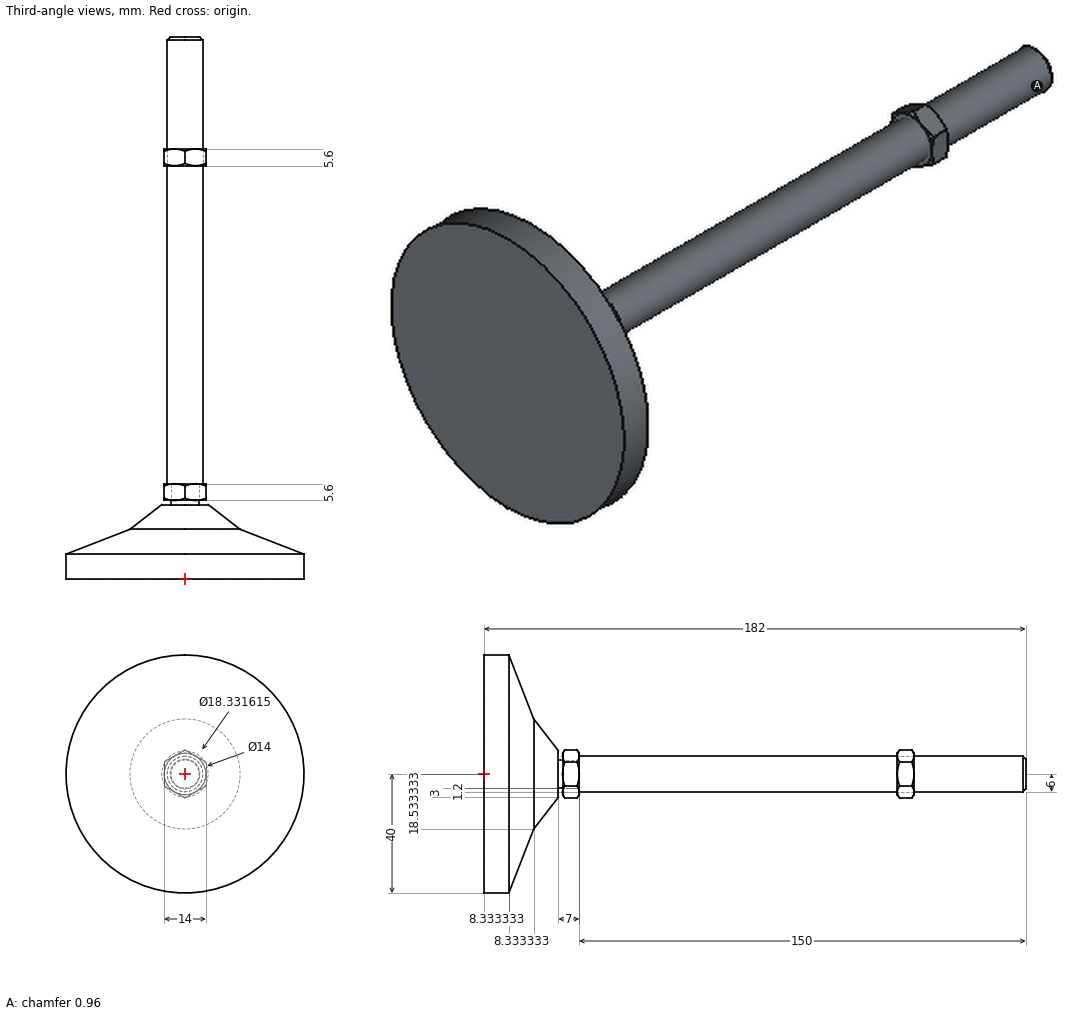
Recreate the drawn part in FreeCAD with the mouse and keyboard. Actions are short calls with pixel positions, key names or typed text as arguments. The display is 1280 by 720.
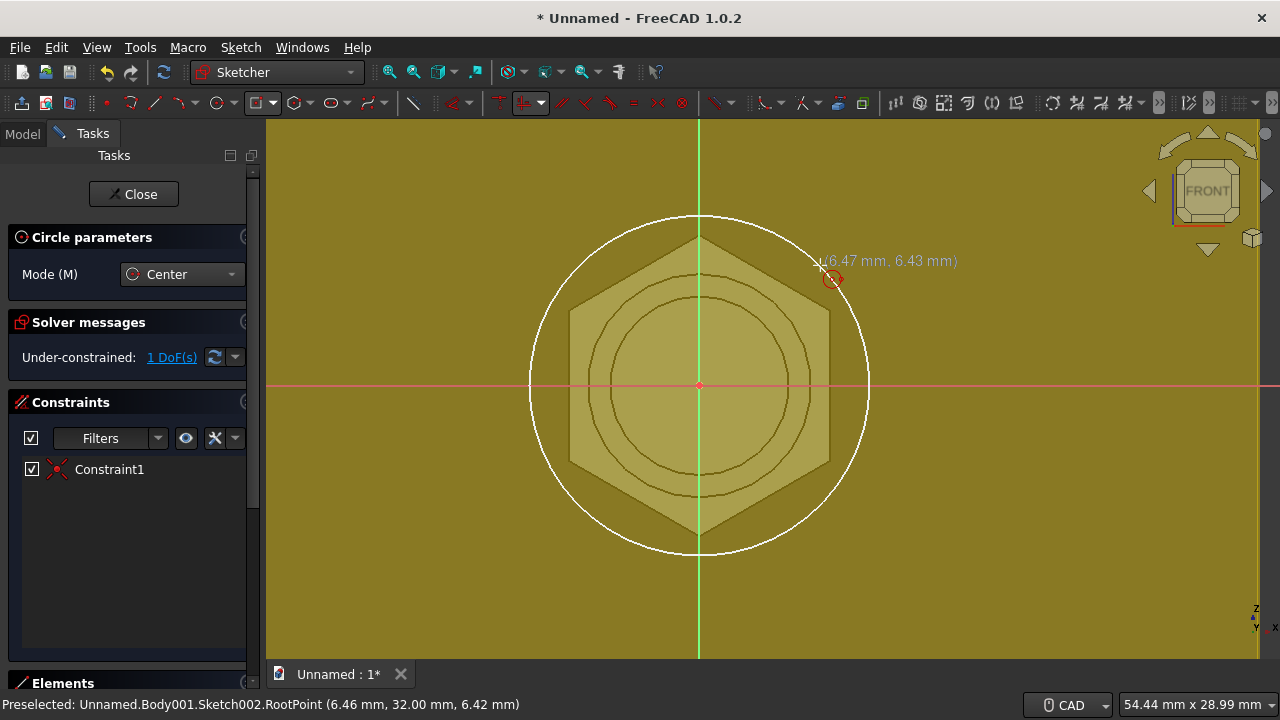
click(699, 386)
click(792, 294)
key(Escape)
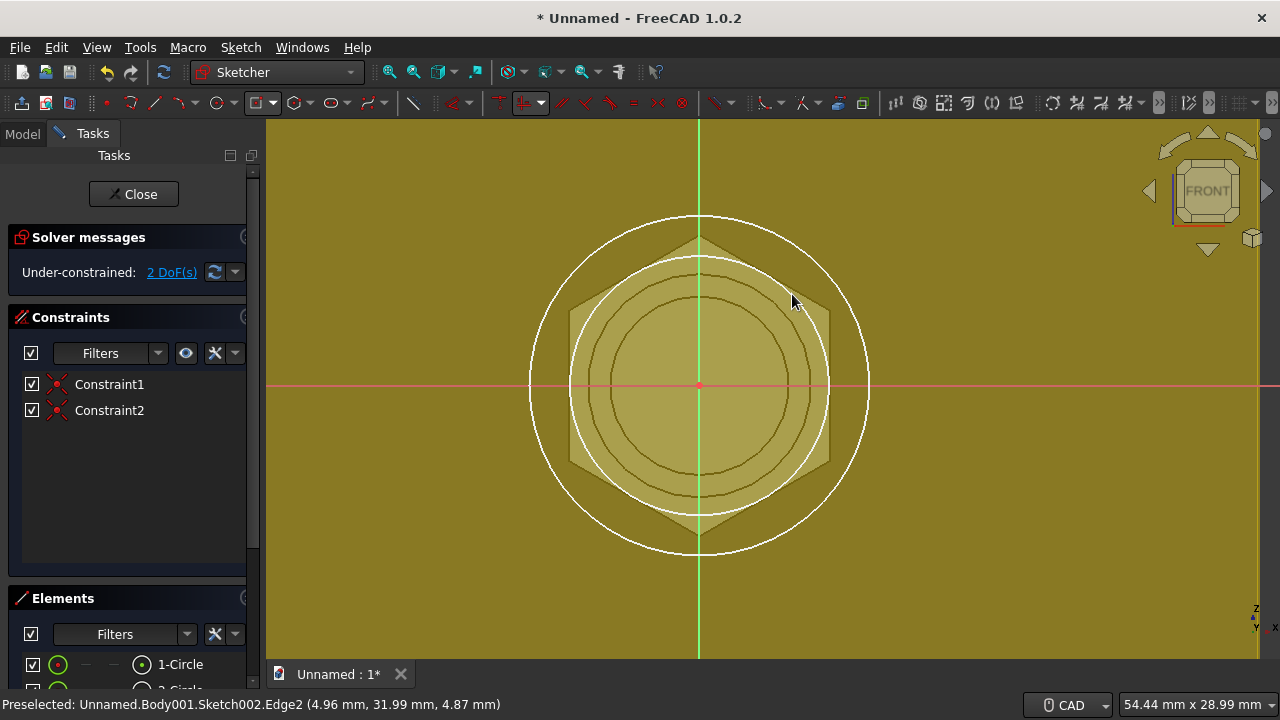
click(452, 104)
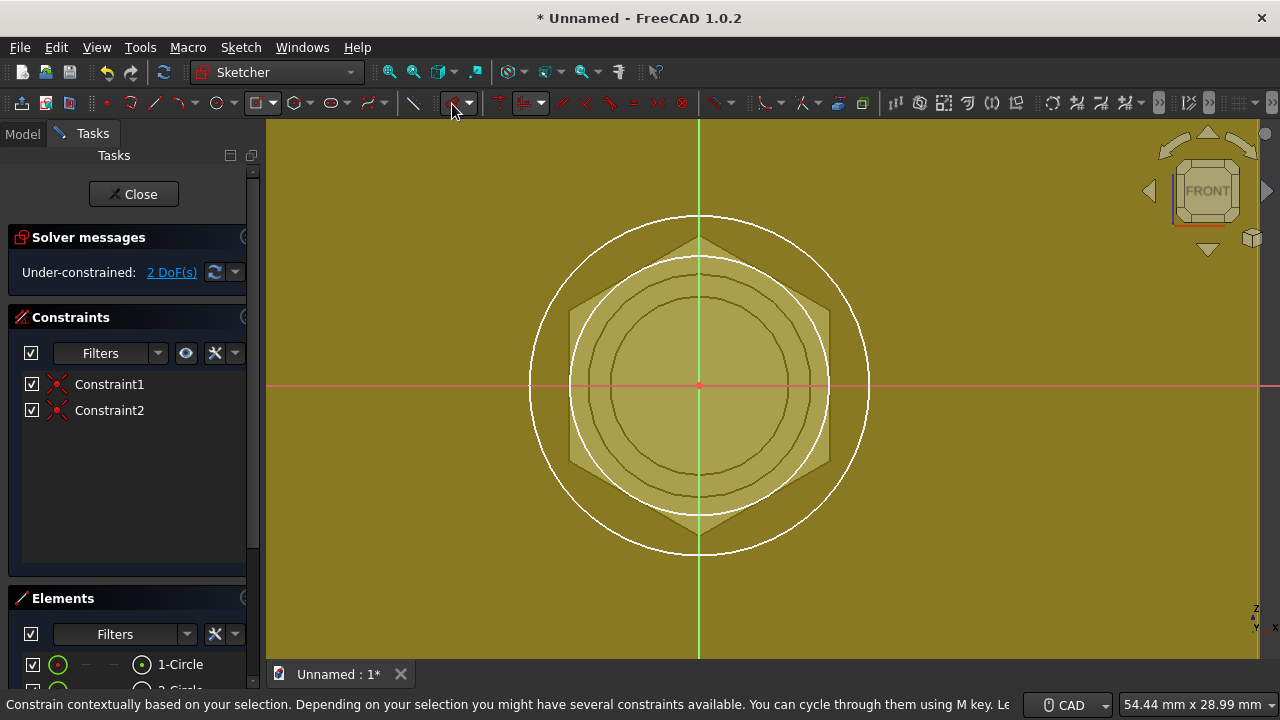
click(819, 265)
click(842, 242)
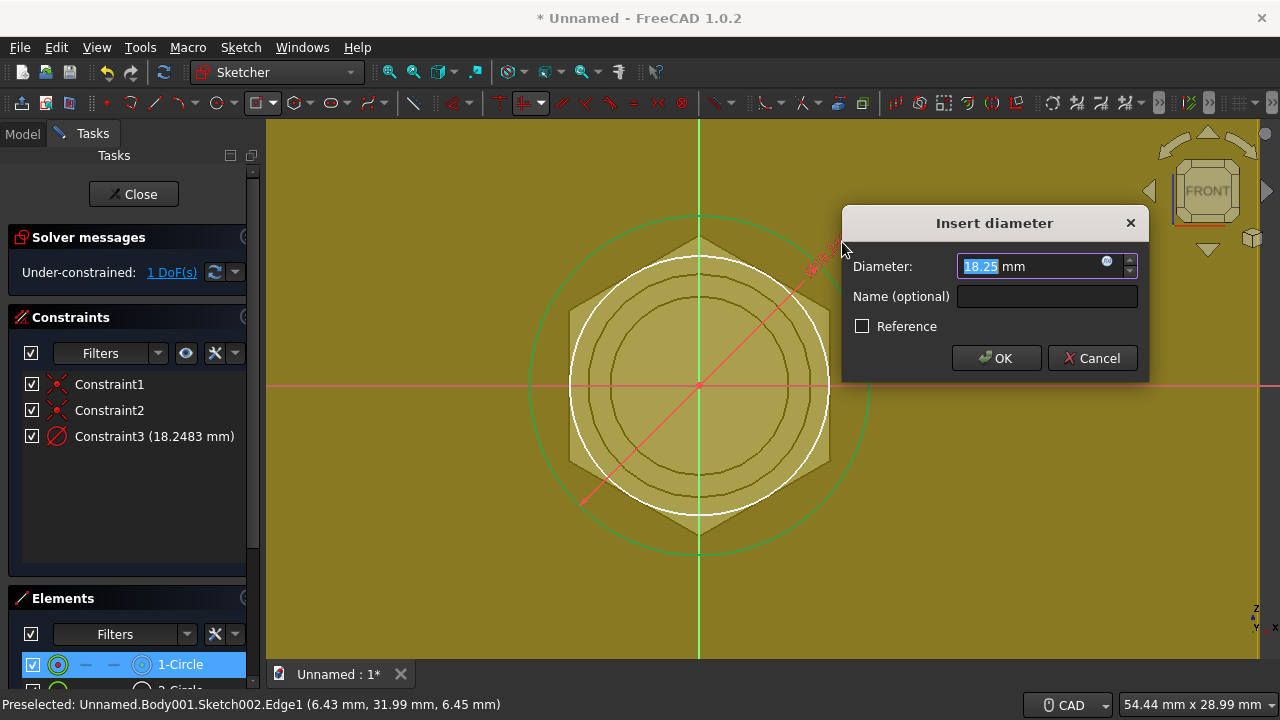
text(18.331615)
key(Return)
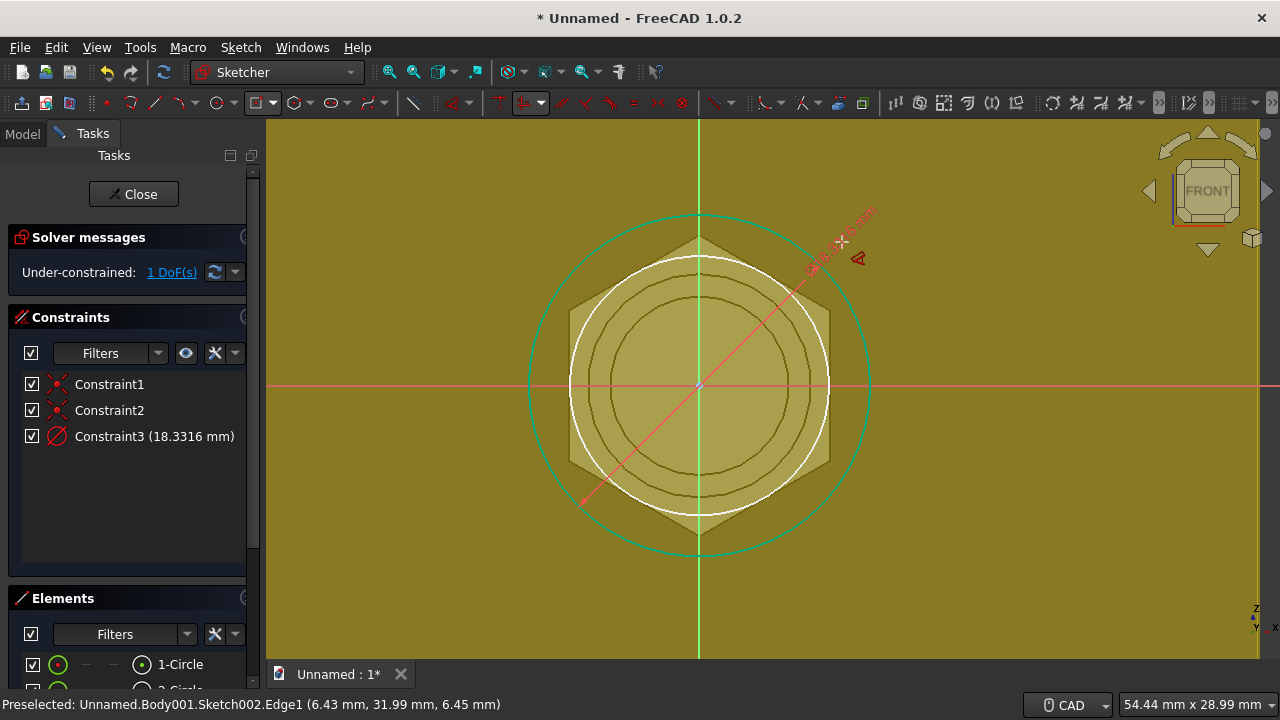
click(791, 294)
click(877, 334)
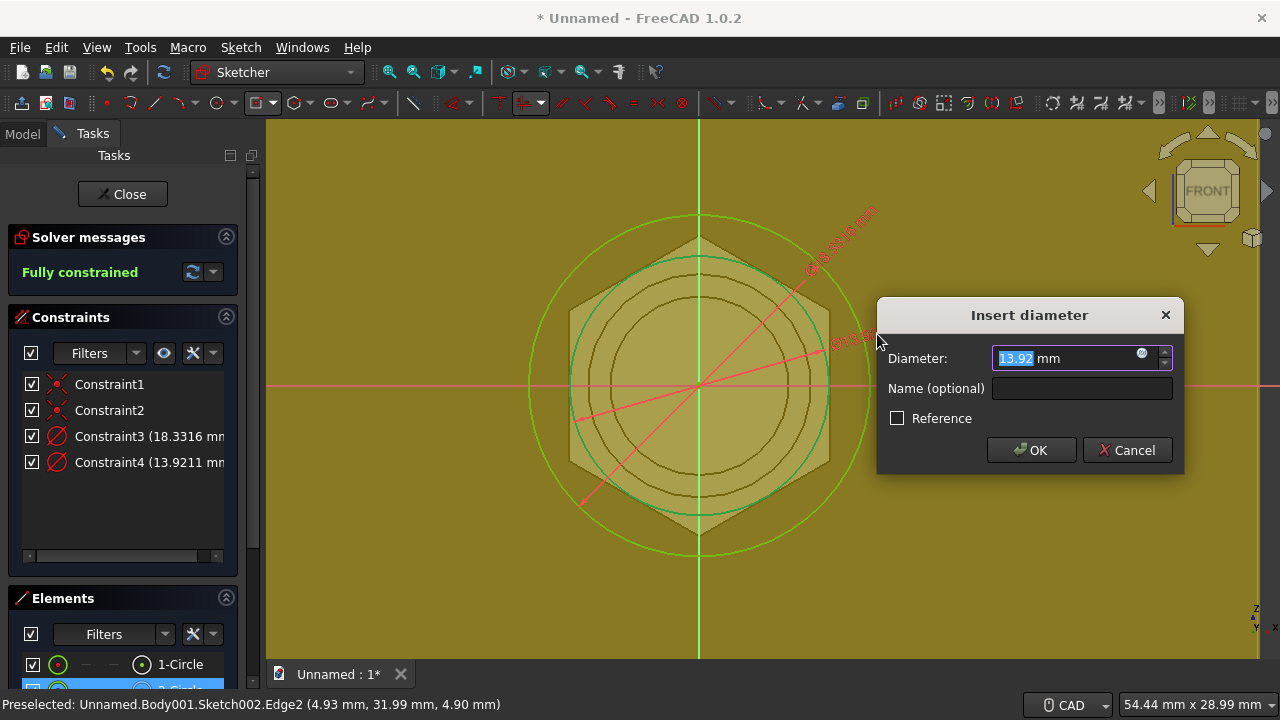
text(14)
key(Return)
key(Escape)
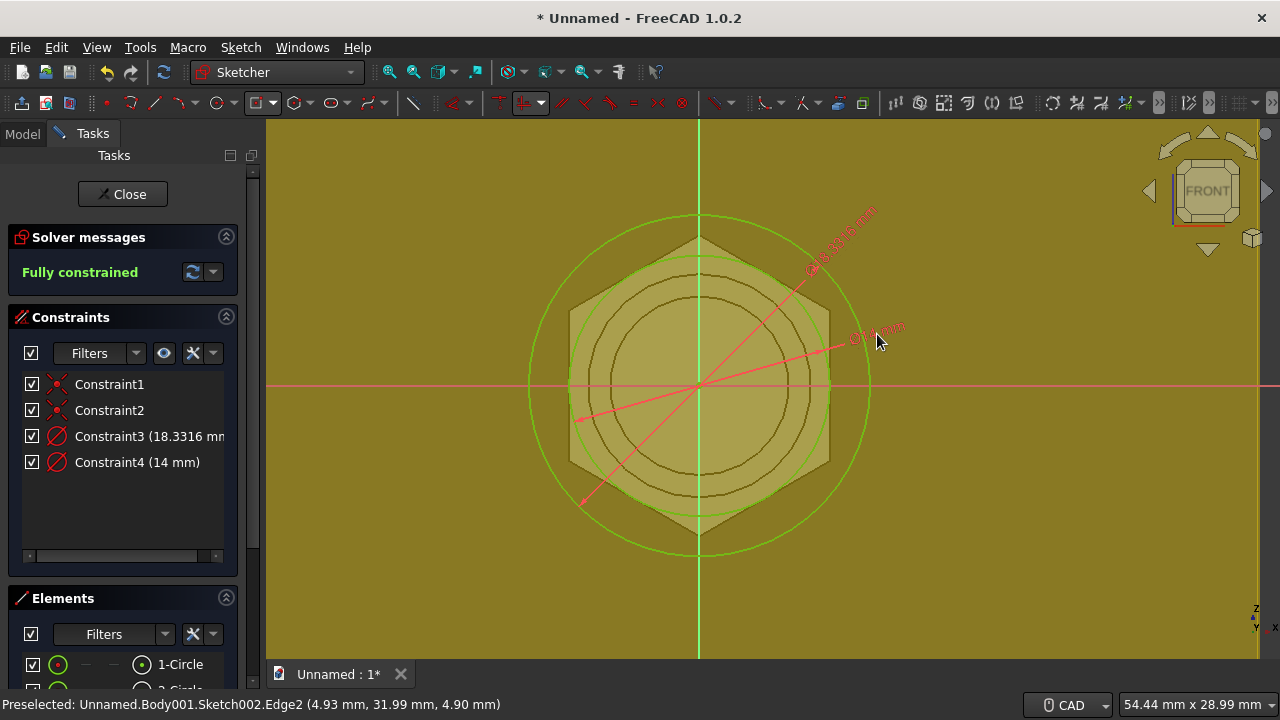
click(123, 194)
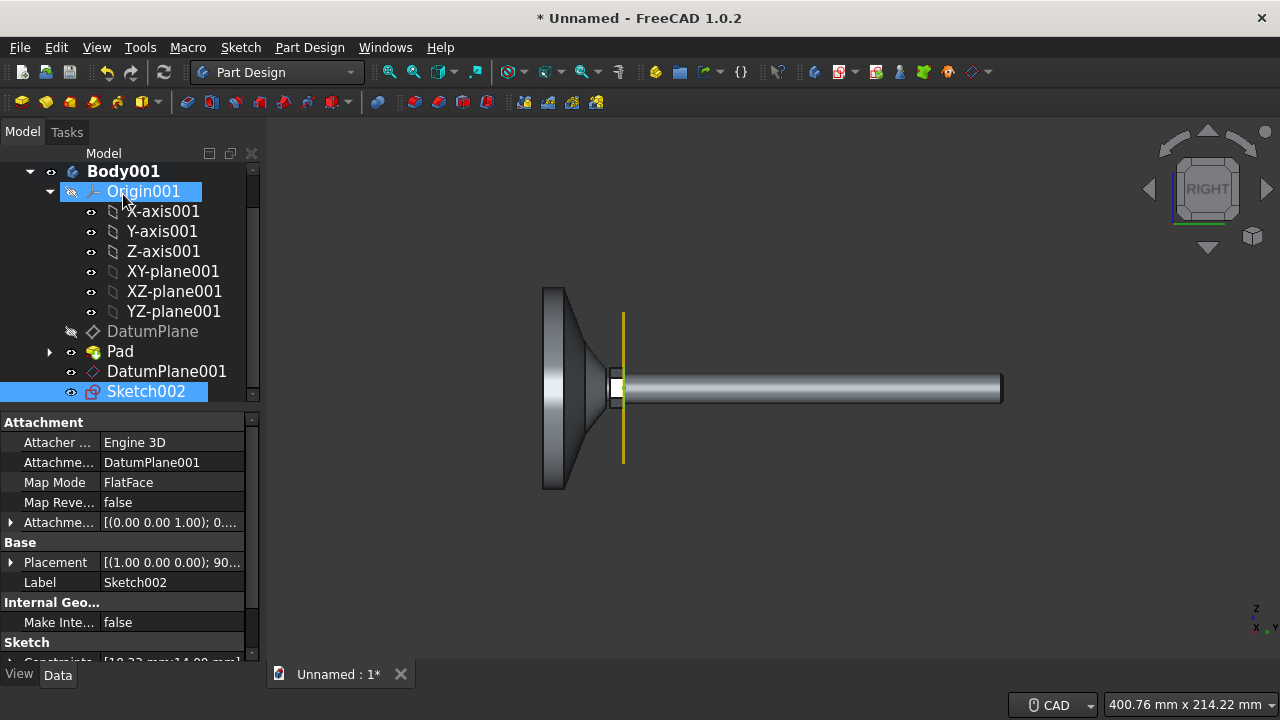
click(188, 102)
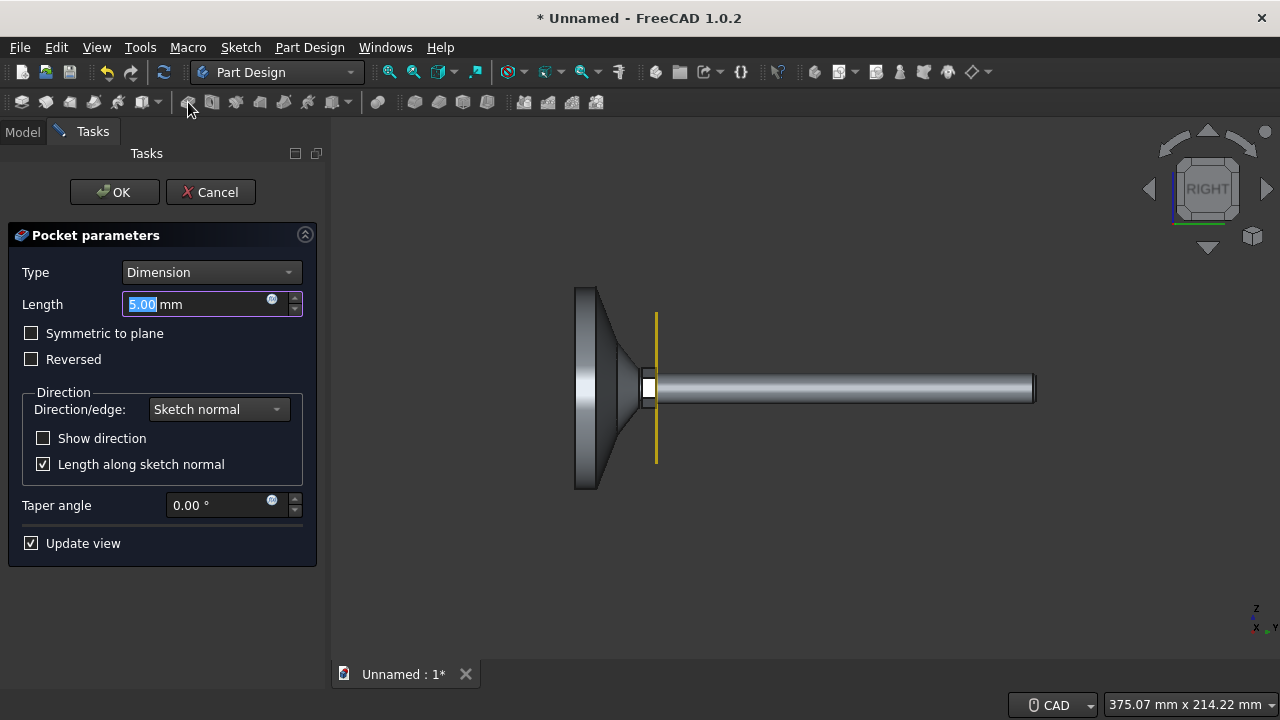
text(5.6)
key(Tab)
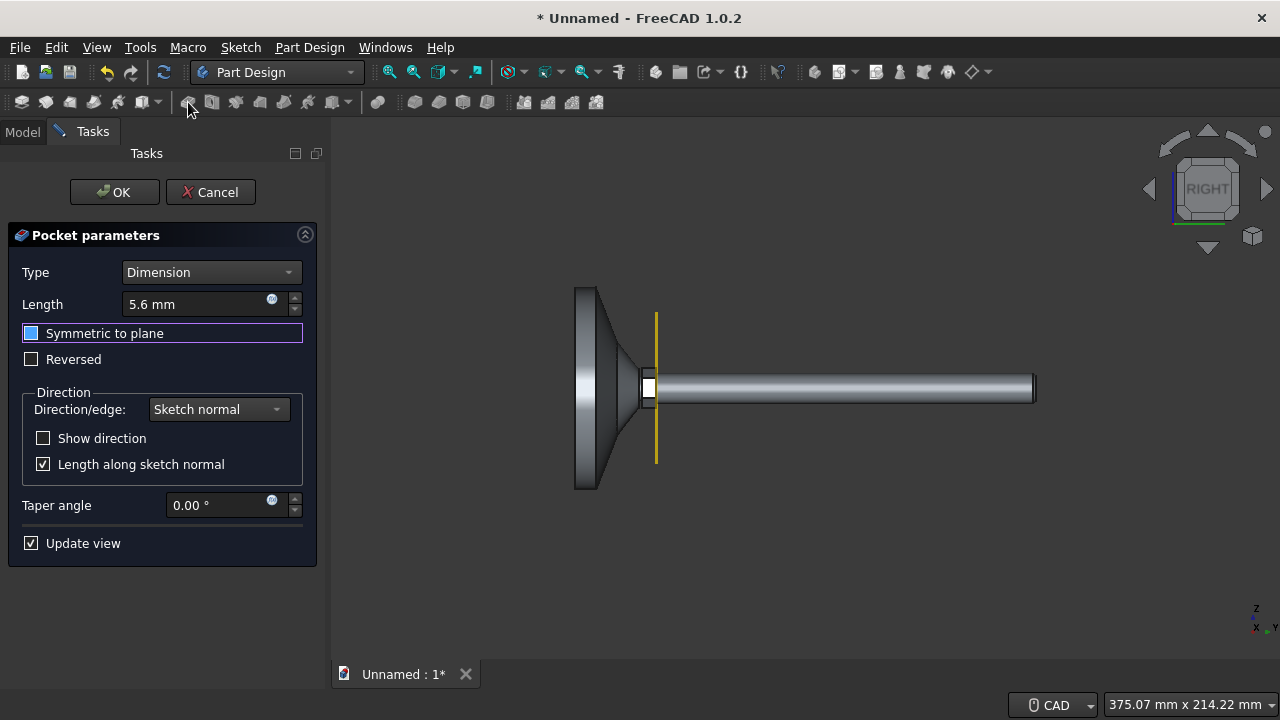
click(30, 359)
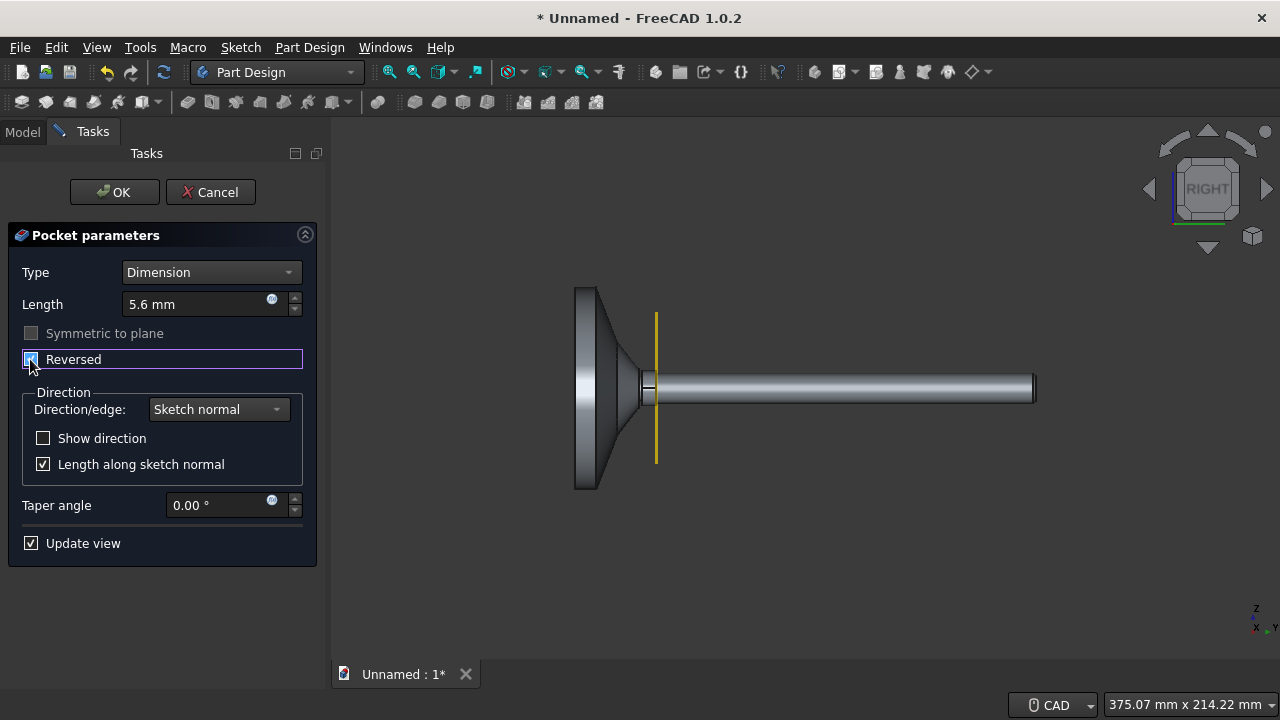
triple_click(226, 505)